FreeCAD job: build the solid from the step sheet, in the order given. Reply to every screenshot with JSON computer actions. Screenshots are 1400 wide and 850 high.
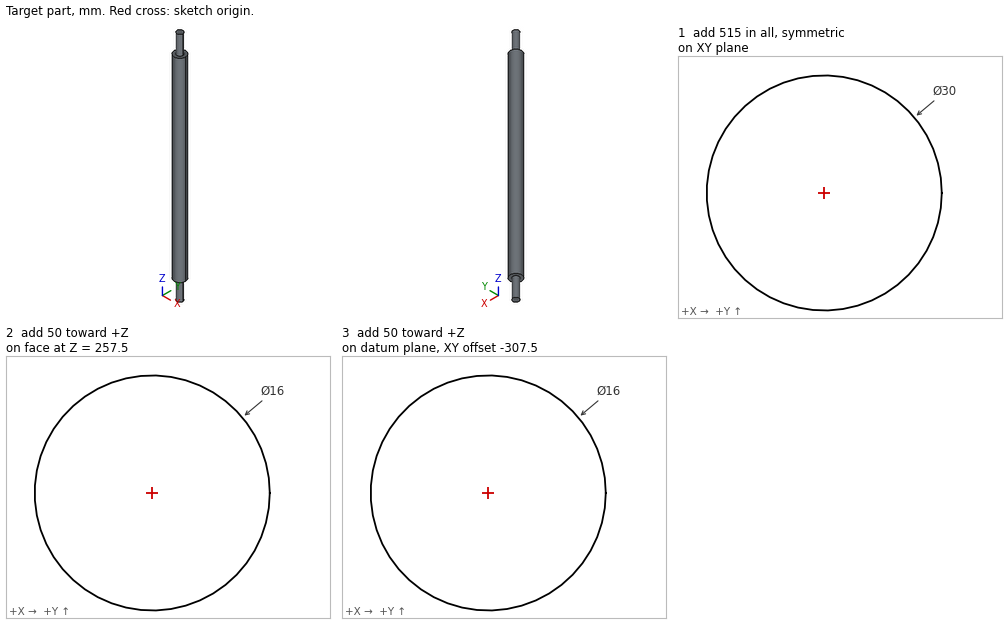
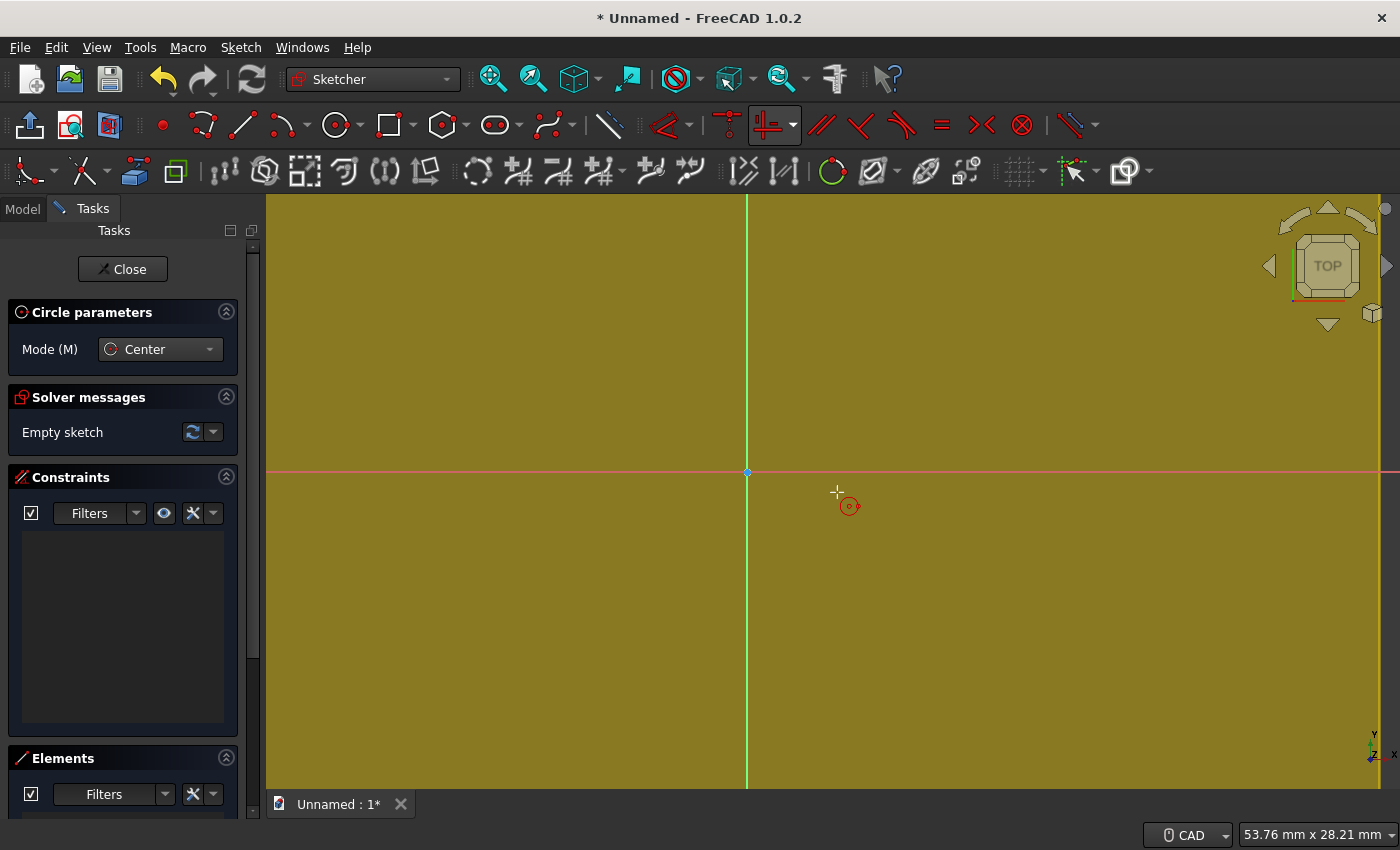
{"action": "left_click", "coordinate": [747, 472]}
{"action": "mouse_move", "coordinate": [866, 353]}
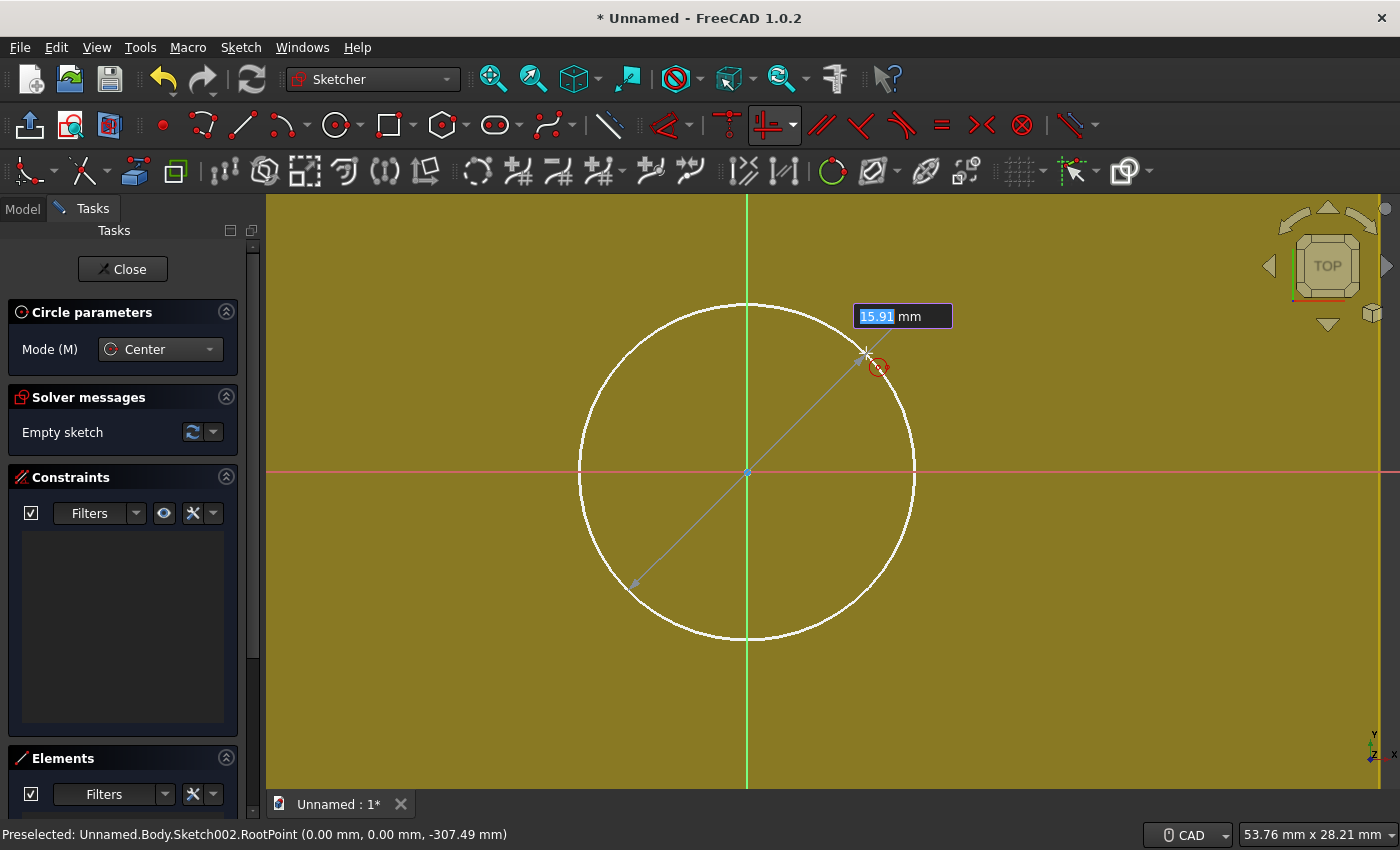
{"action": "type", "text": "16"}
{"action": "key", "text": "Return"}
{"action": "key", "text": "Escape"}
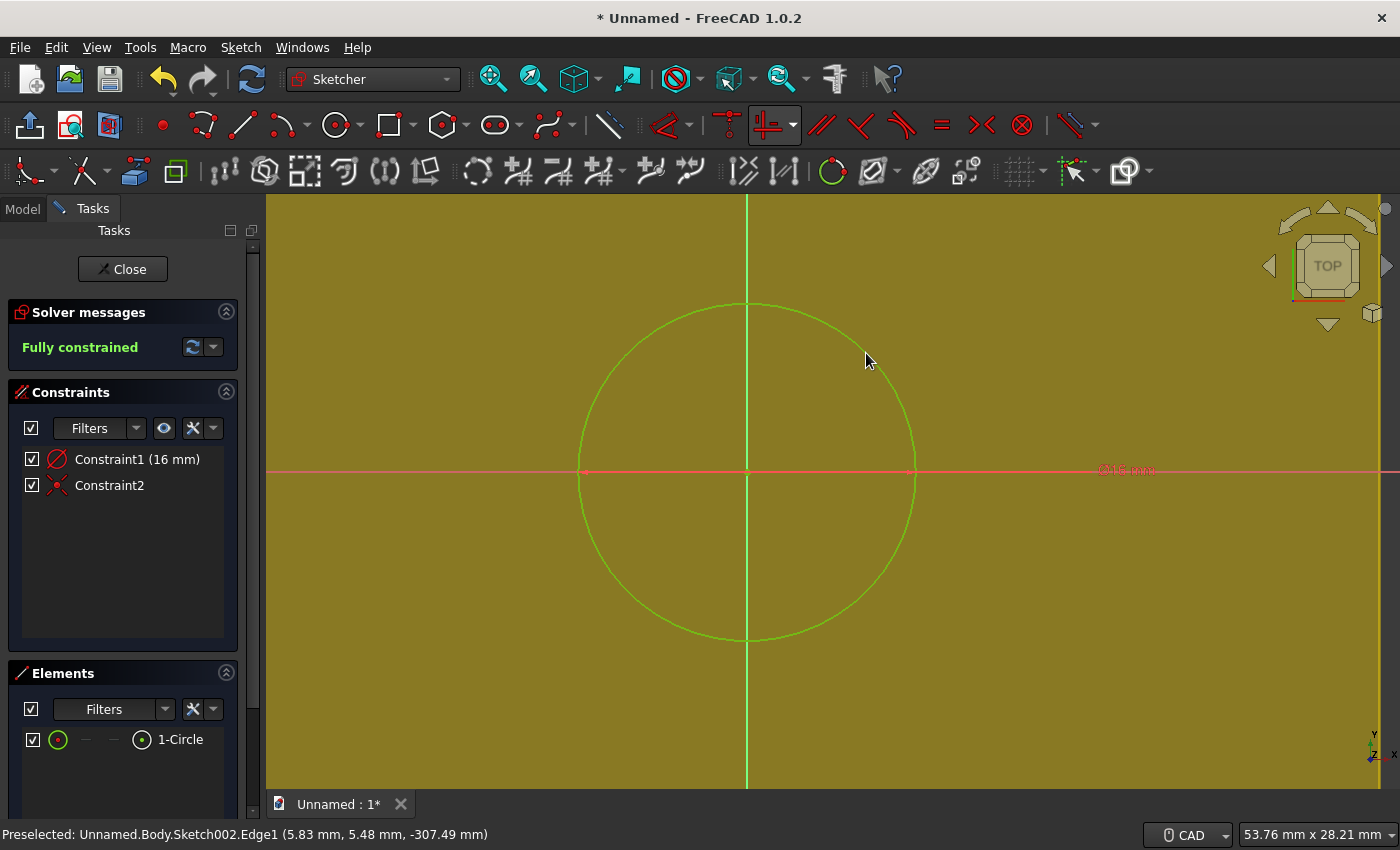
{"action": "left_click", "coordinate": [123, 269]}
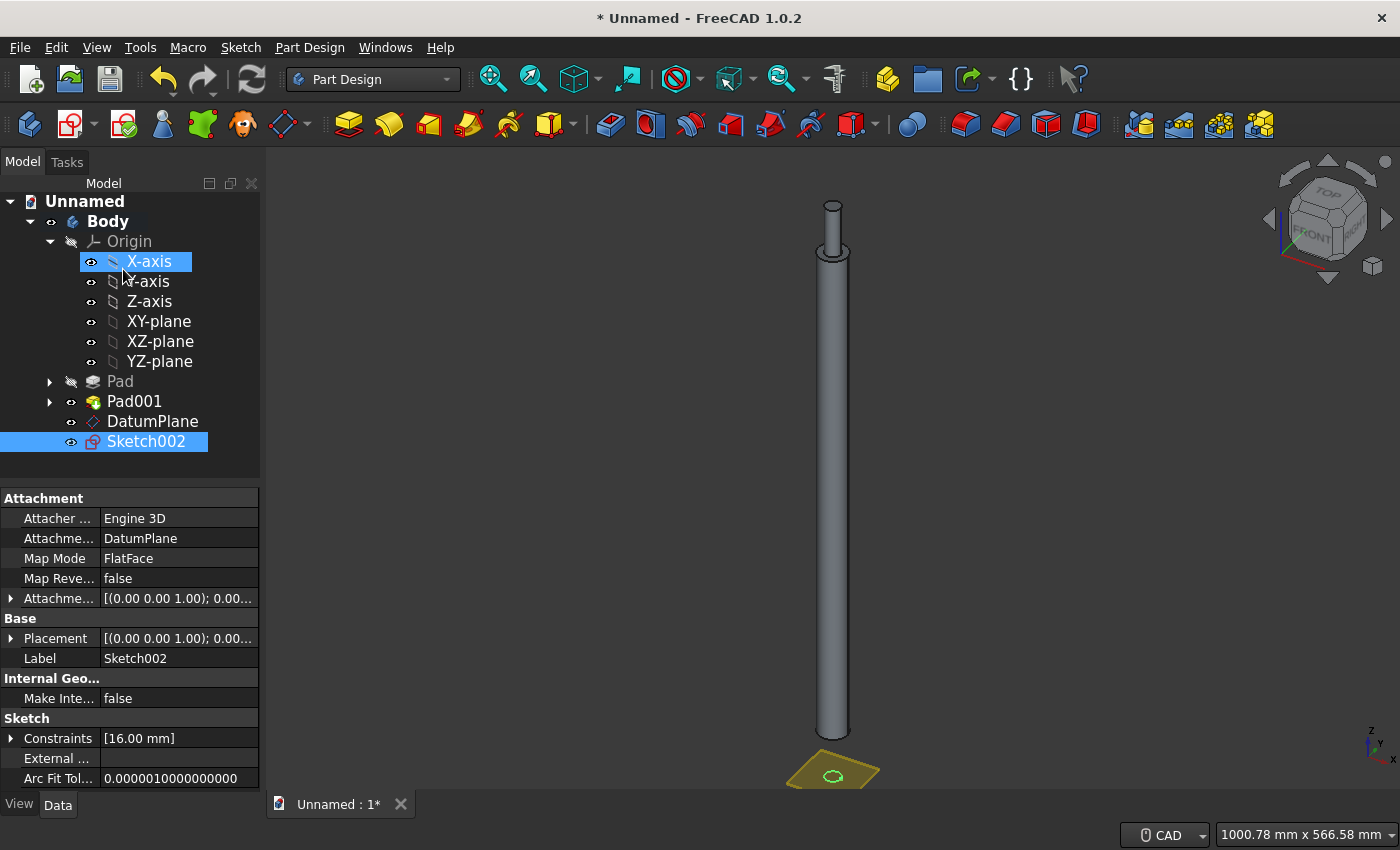
{"action": "left_click", "coordinate": [350, 124]}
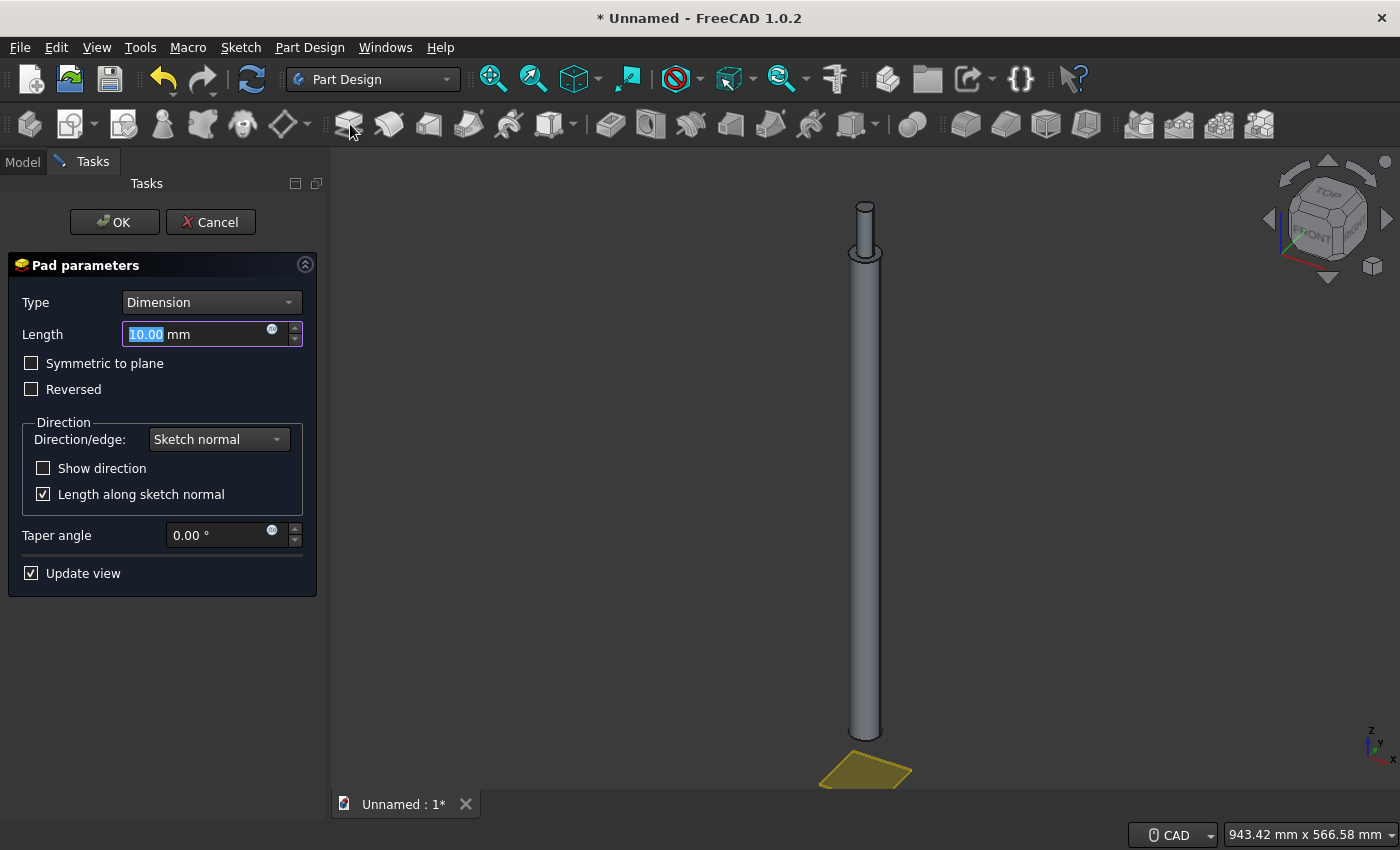
{"action": "type", "text": "50"}
{"action": "key", "text": "Tab"}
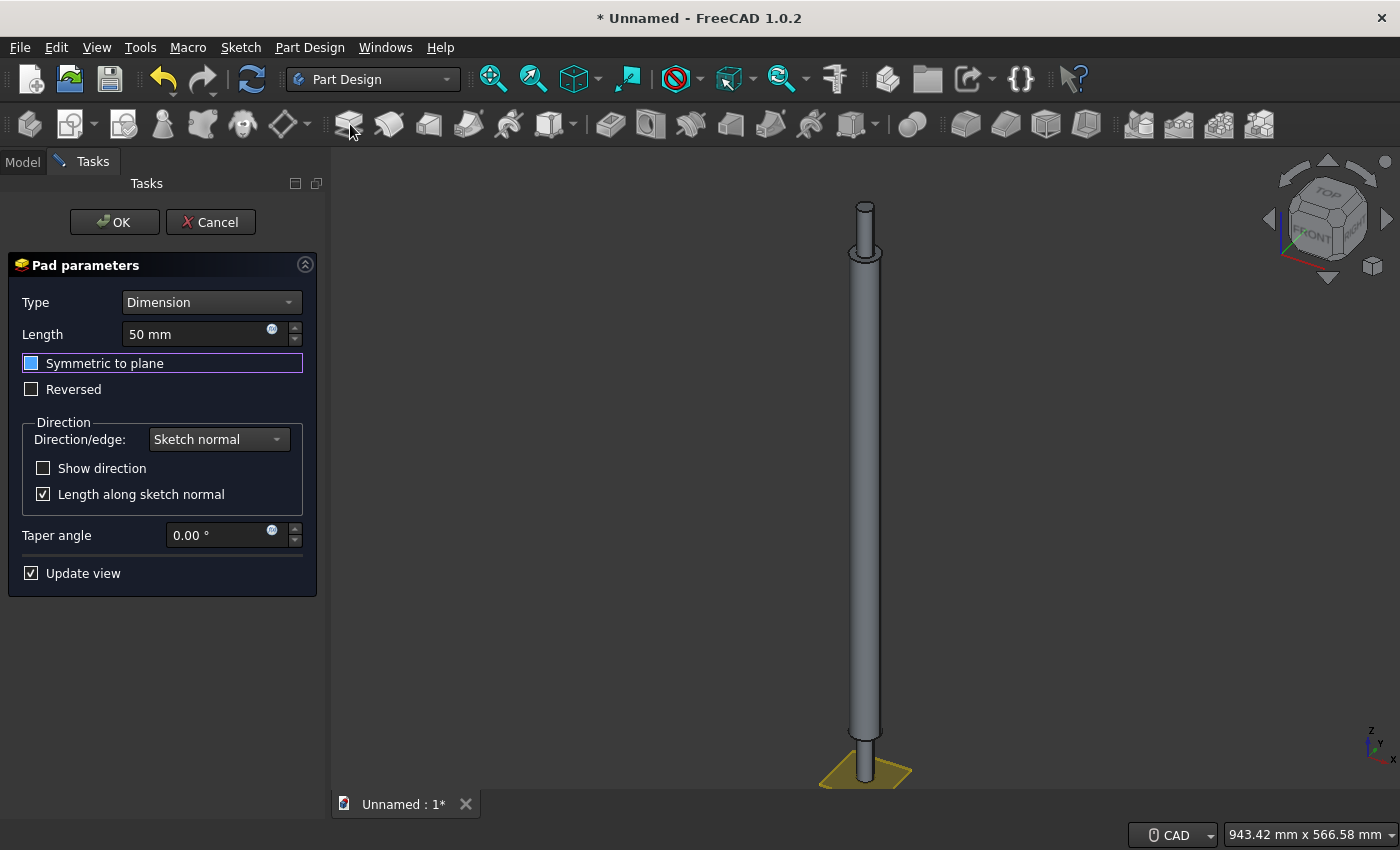
{"action": "left_click", "coordinate": [115, 222]}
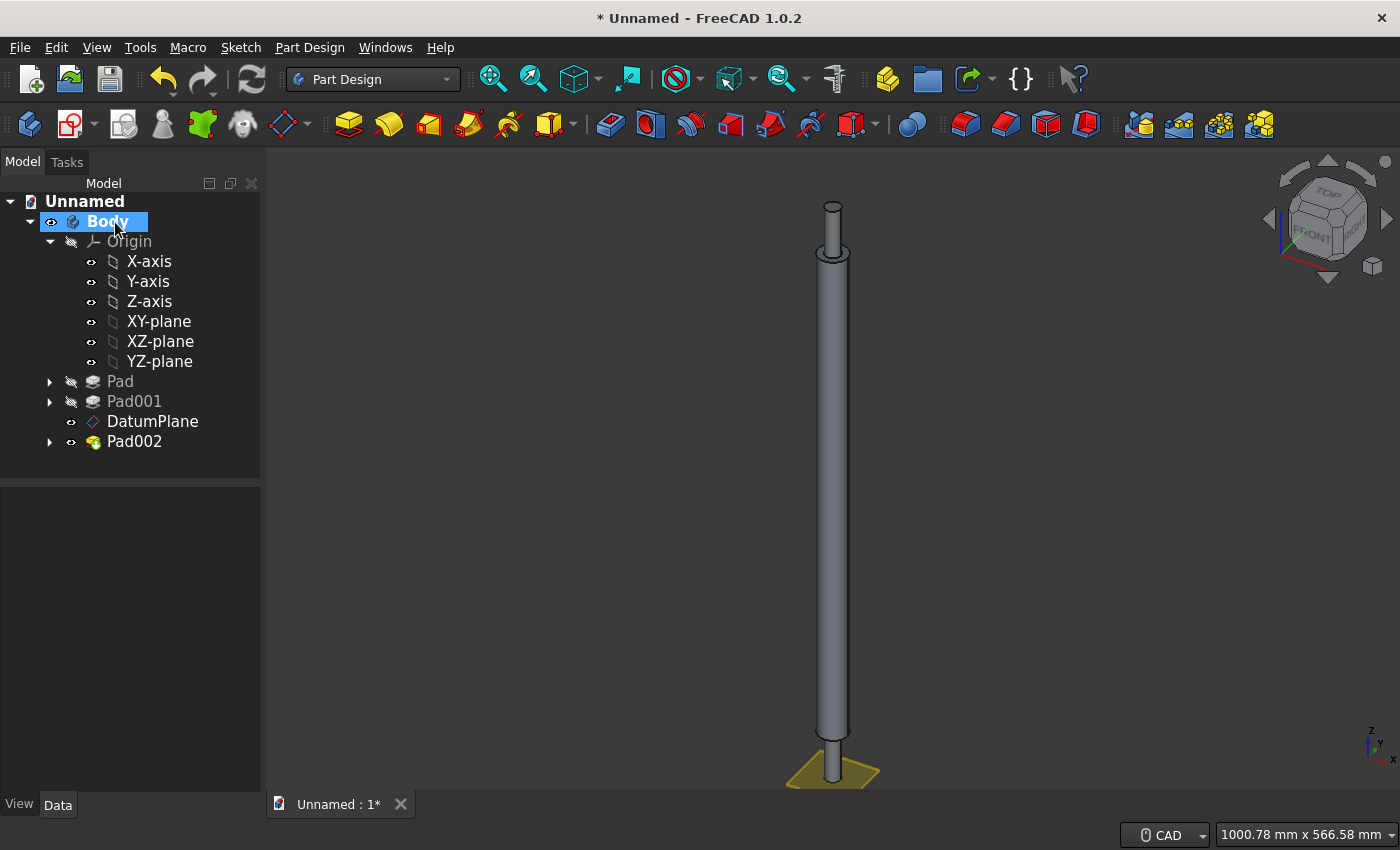
{"action": "left_click", "coordinate": [116, 422]}
{"action": "key", "text": "space"}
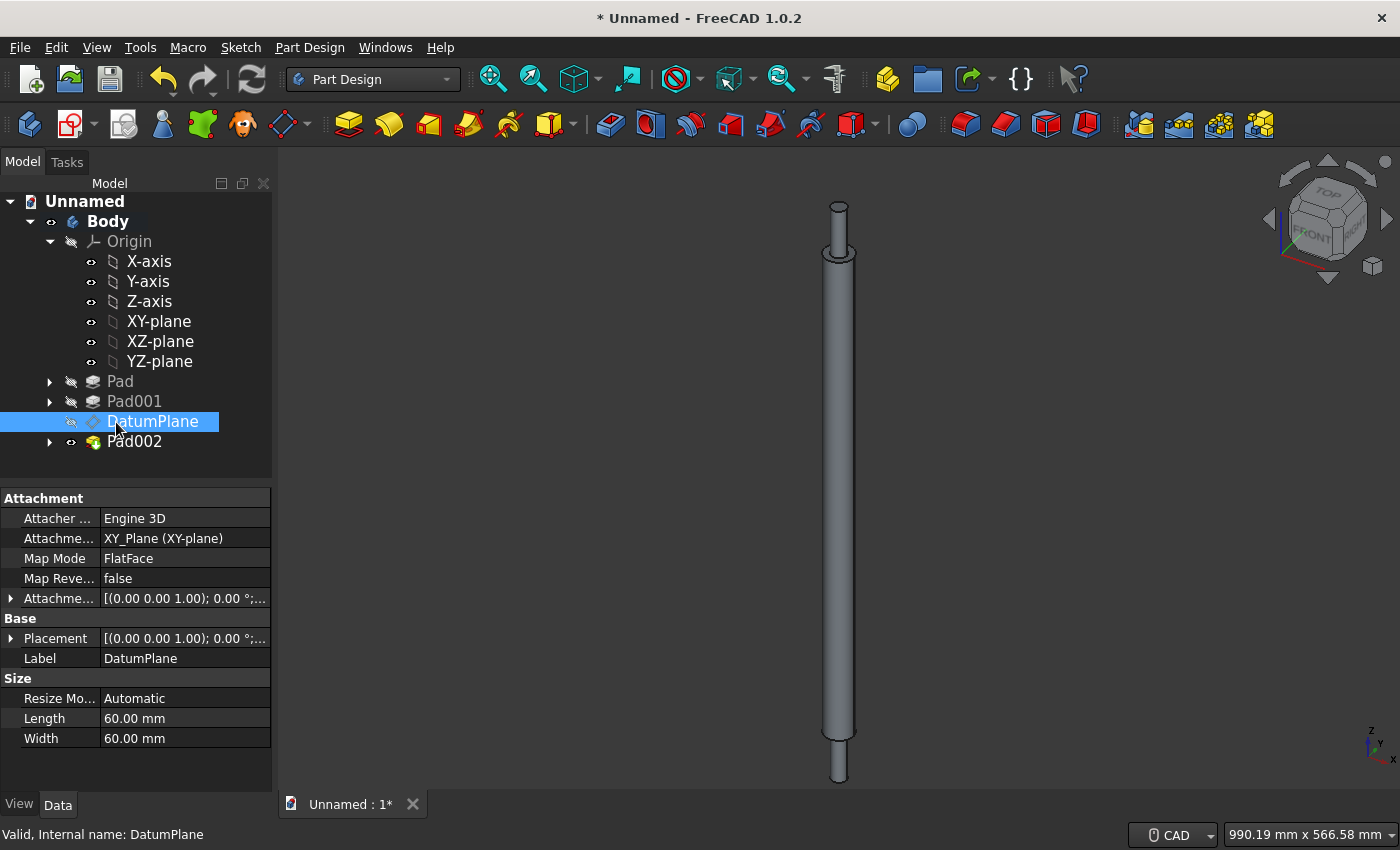
{"action": "key", "text": "0"}